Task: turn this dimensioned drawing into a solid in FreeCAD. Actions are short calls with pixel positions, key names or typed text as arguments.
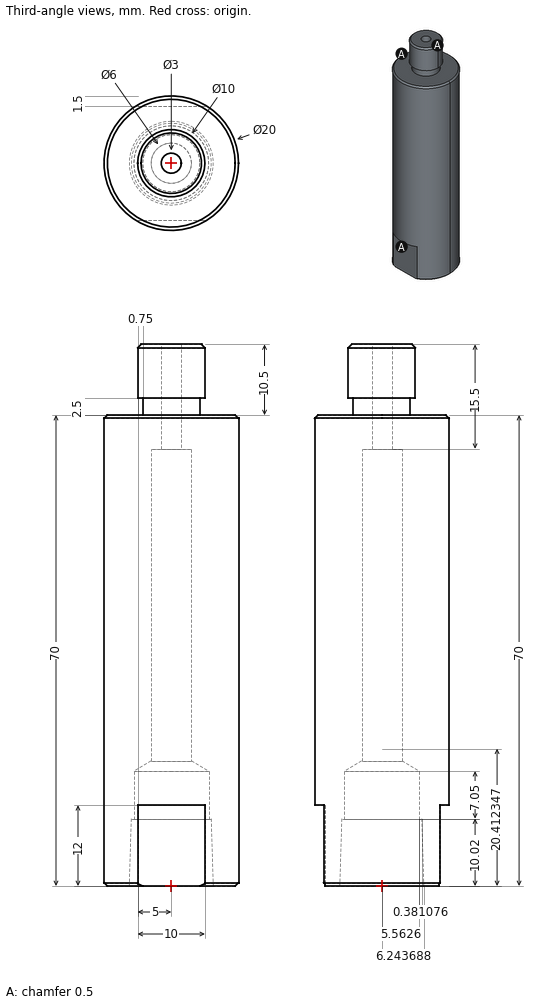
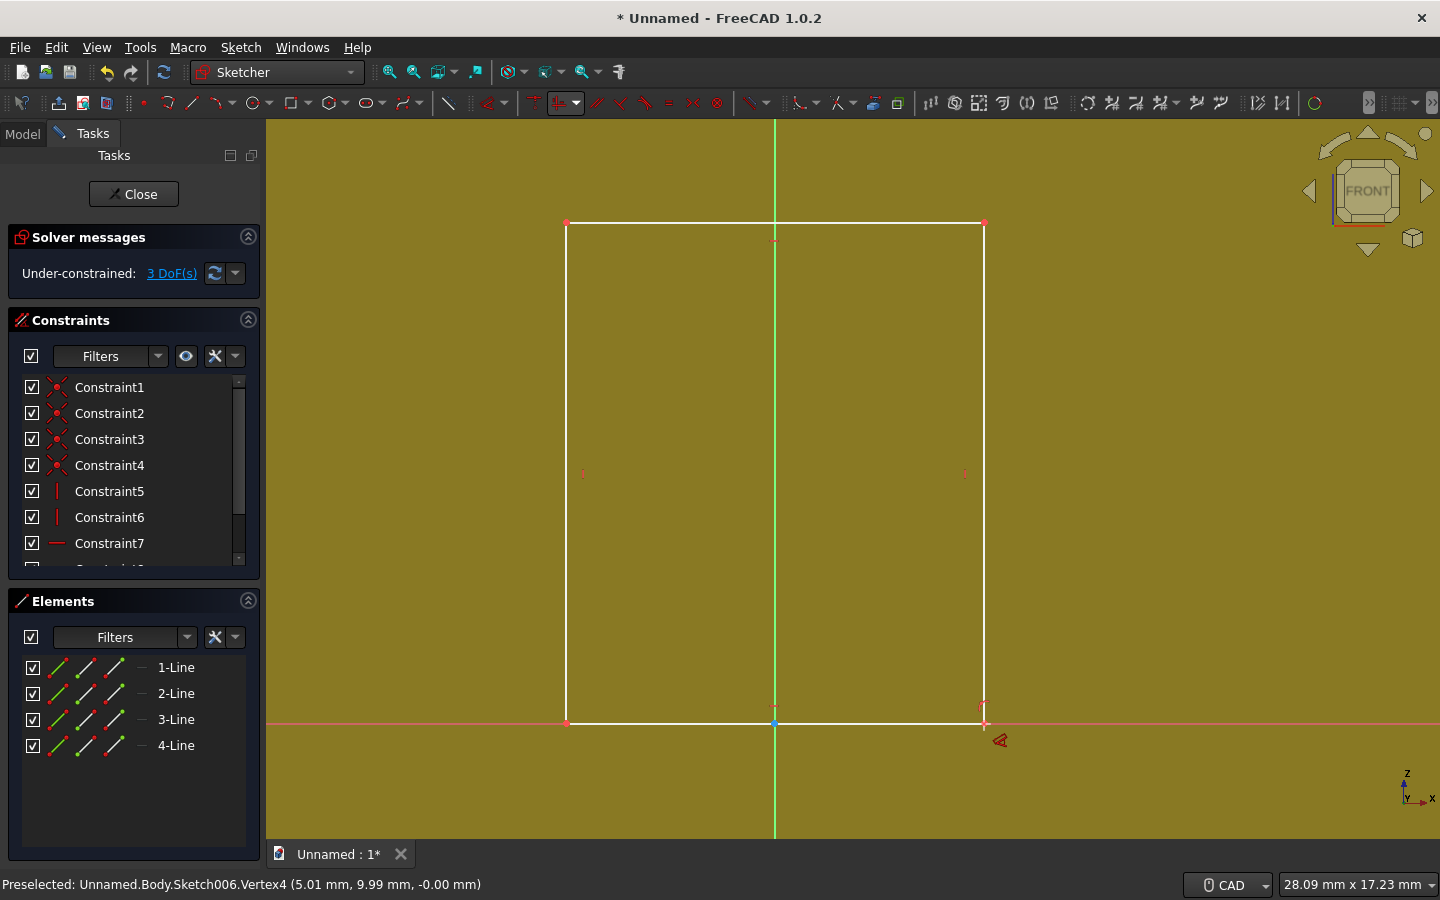
click(566, 373)
click(532, 473)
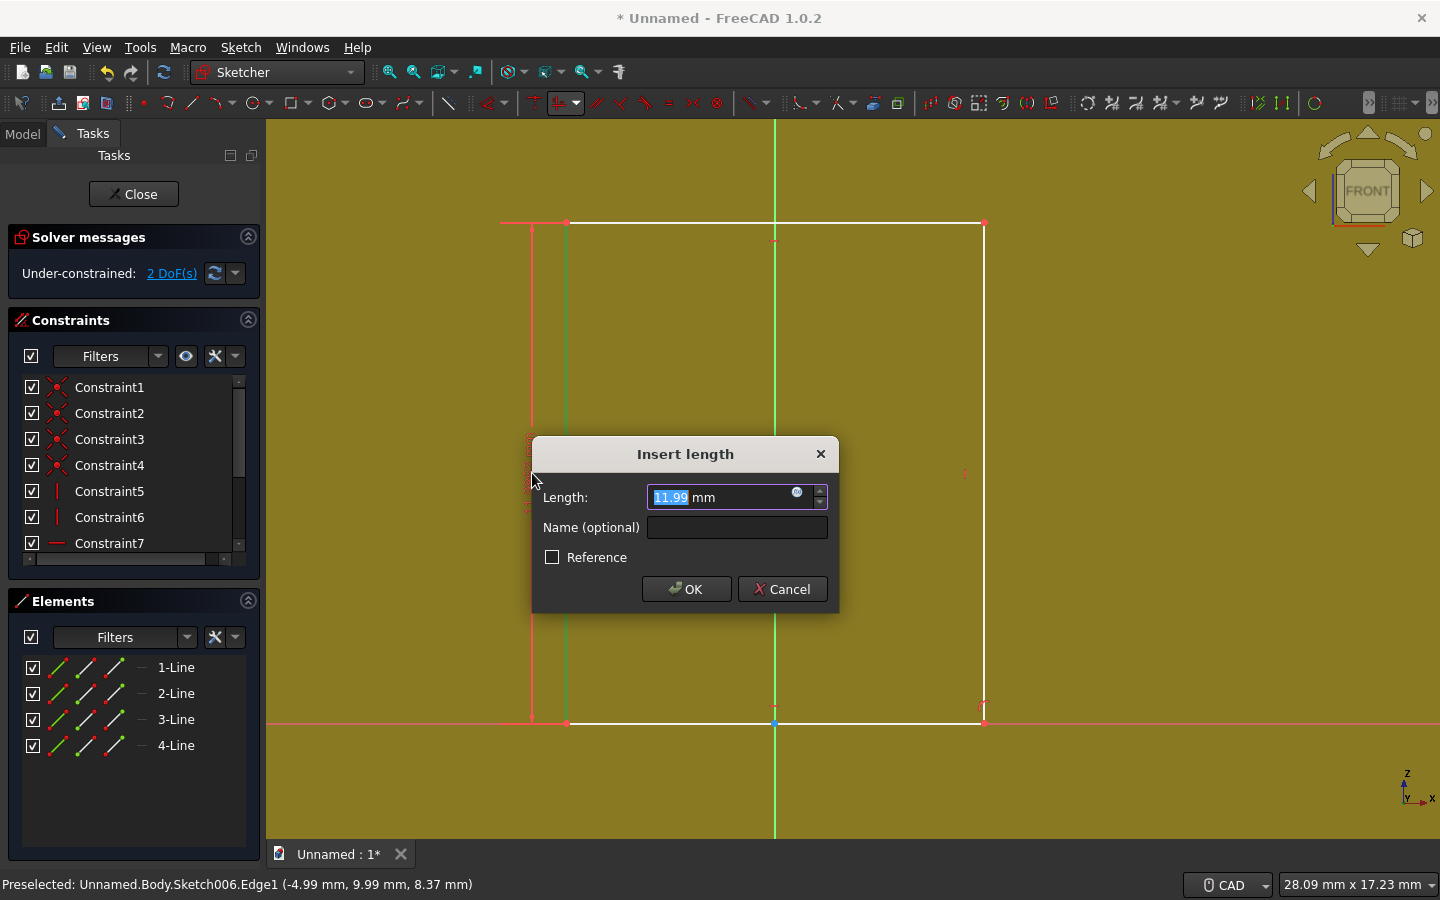
text(12)
key(Return)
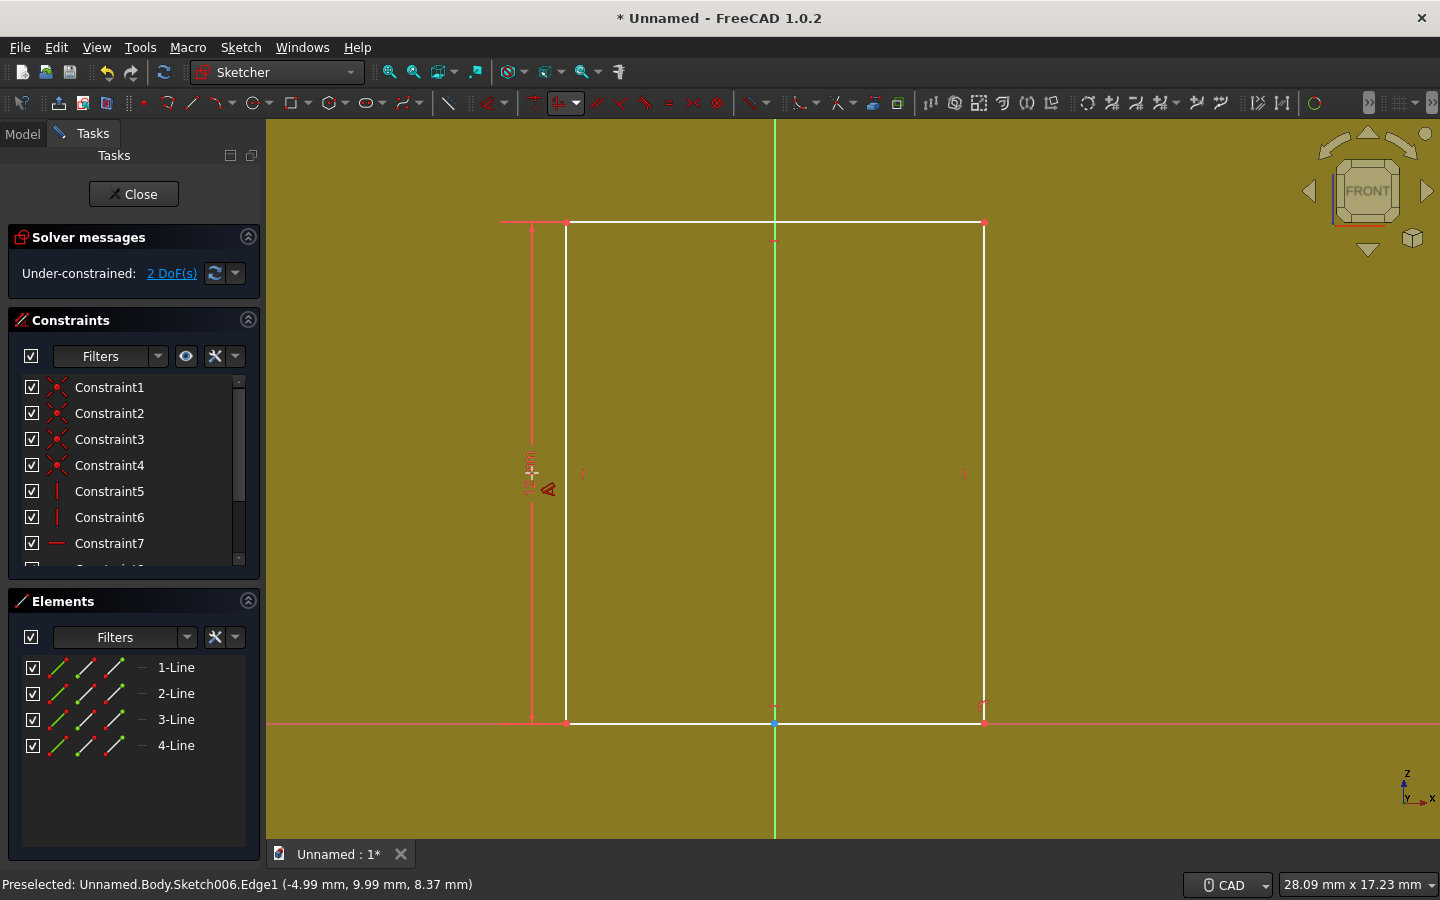
click(691, 724)
click(679, 758)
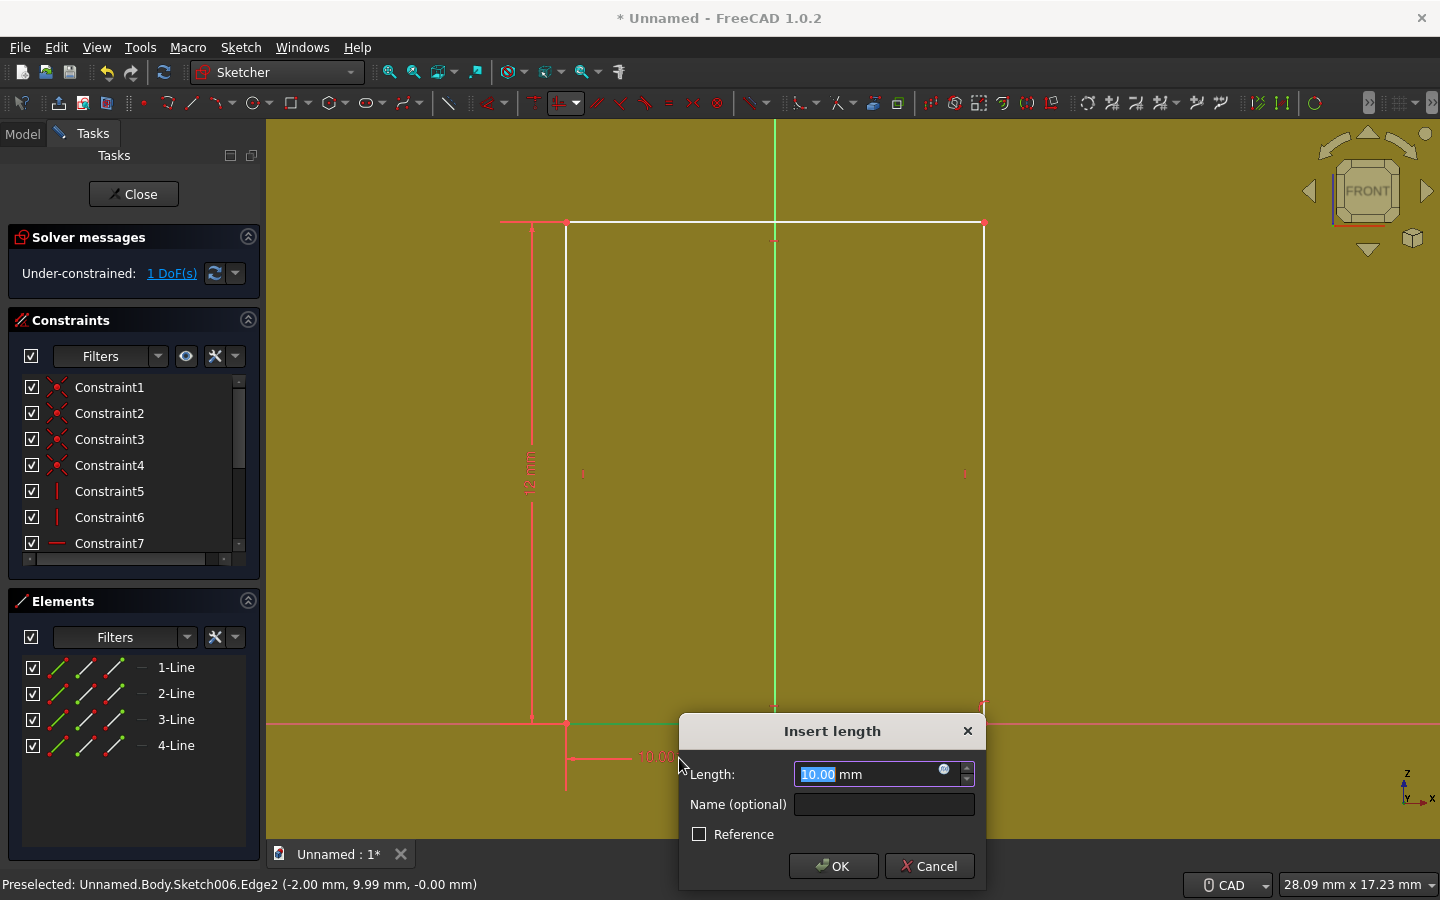
text(10)
key(Return)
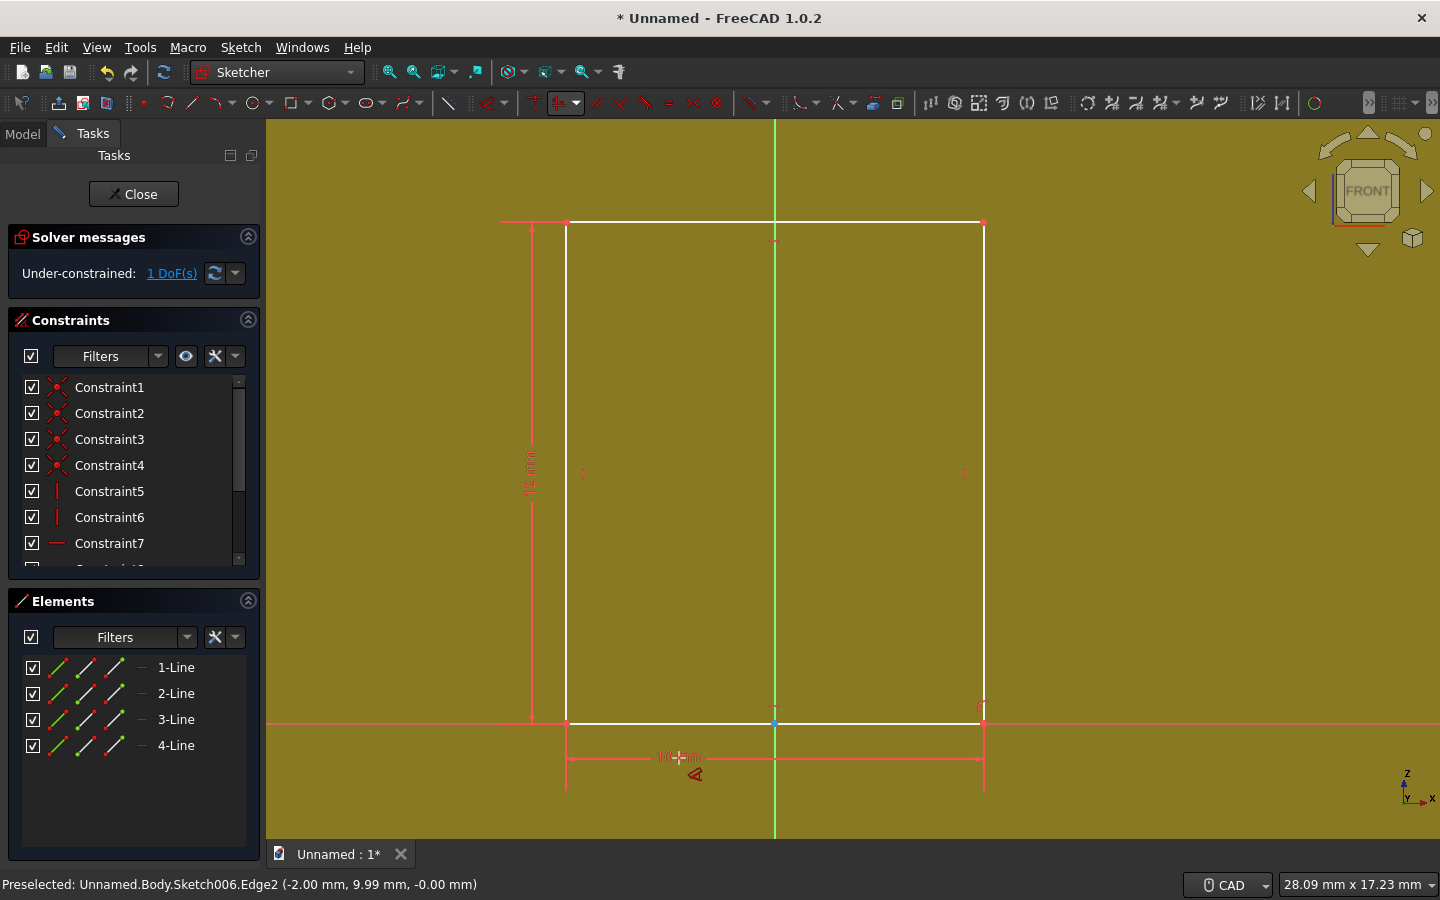
click(566, 222)
click(597, 758)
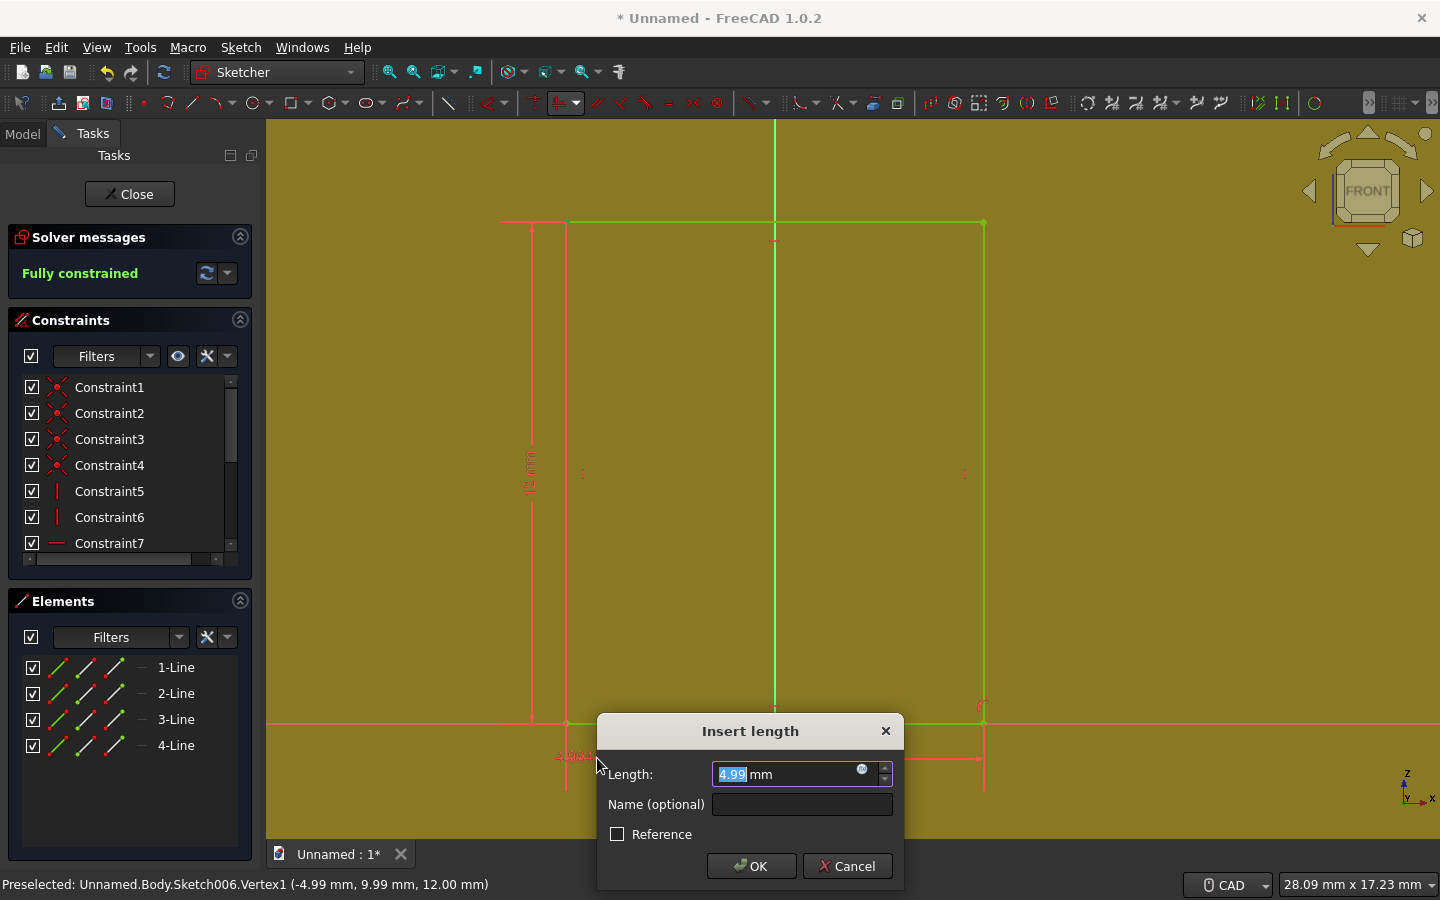
text(5)
key(Return)
key(Escape)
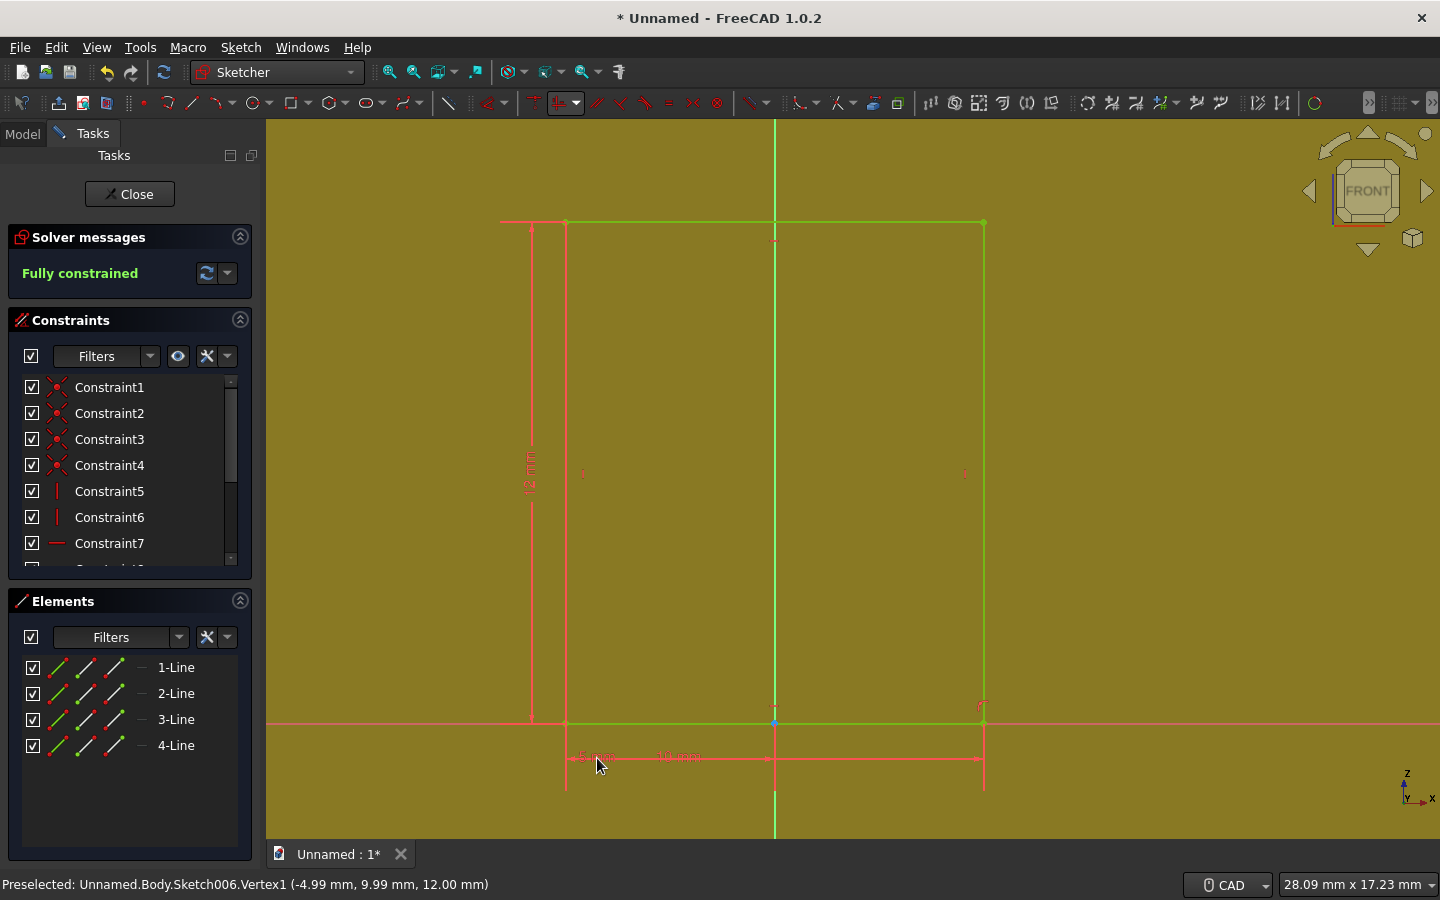
click(130, 194)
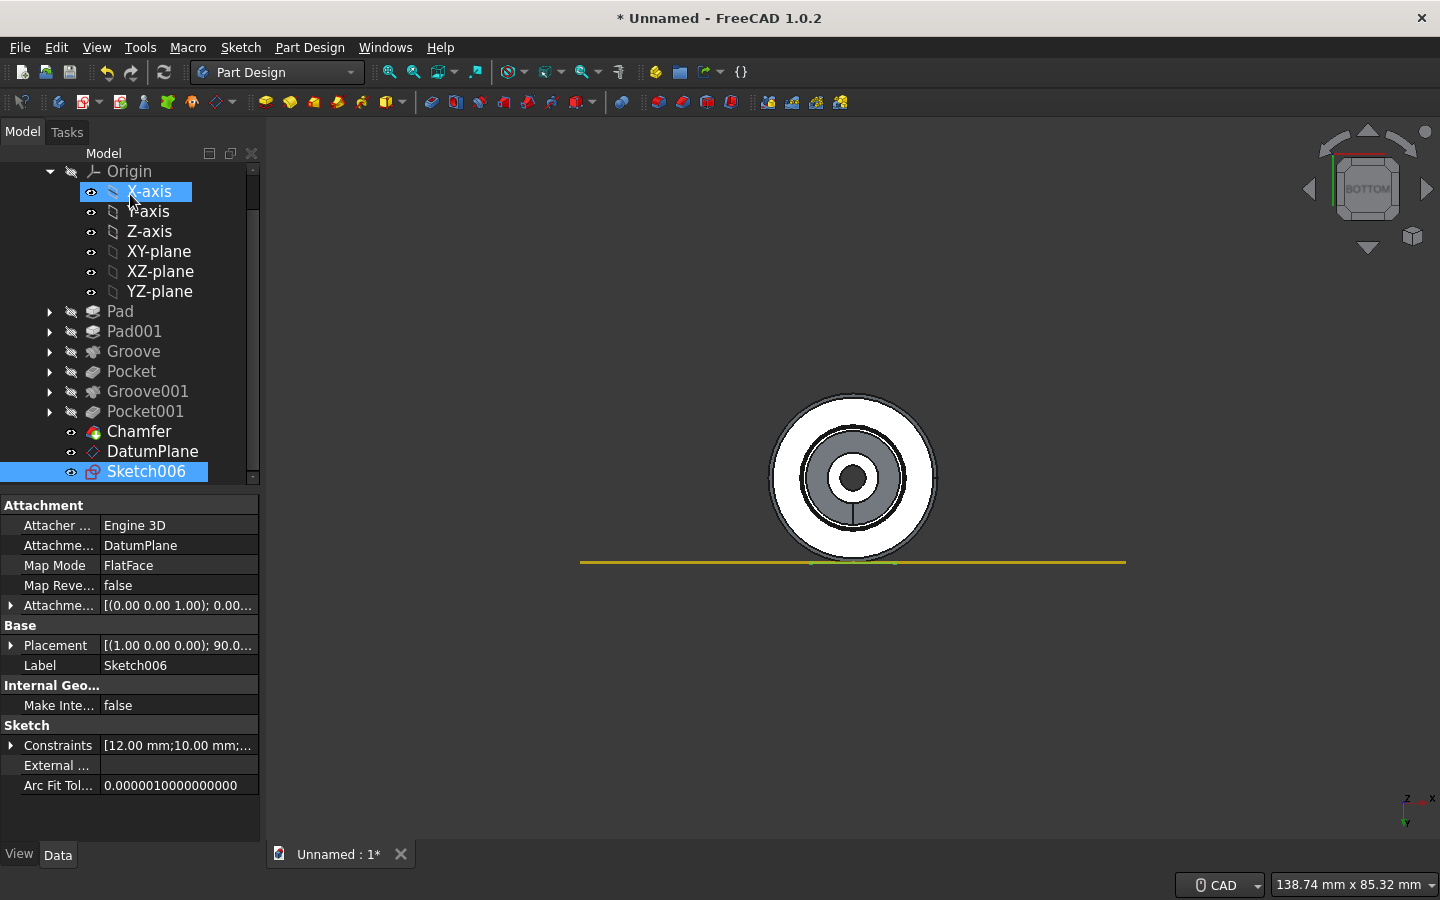
click(432, 102)